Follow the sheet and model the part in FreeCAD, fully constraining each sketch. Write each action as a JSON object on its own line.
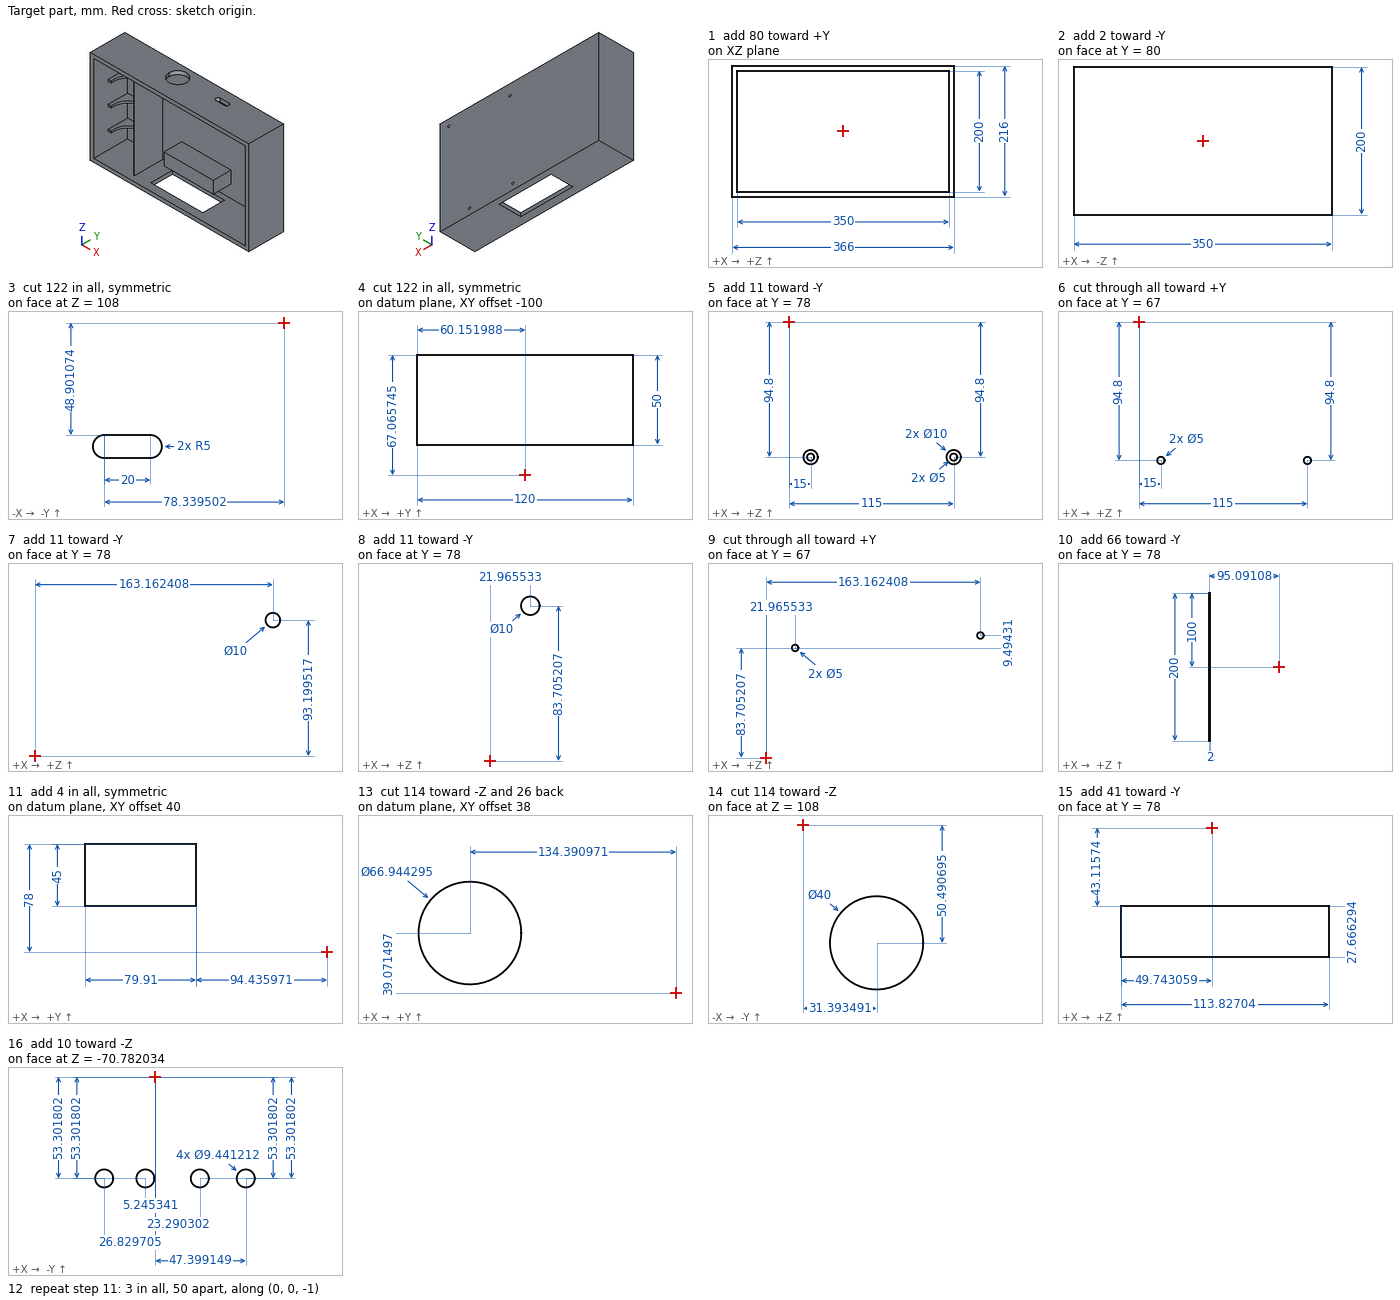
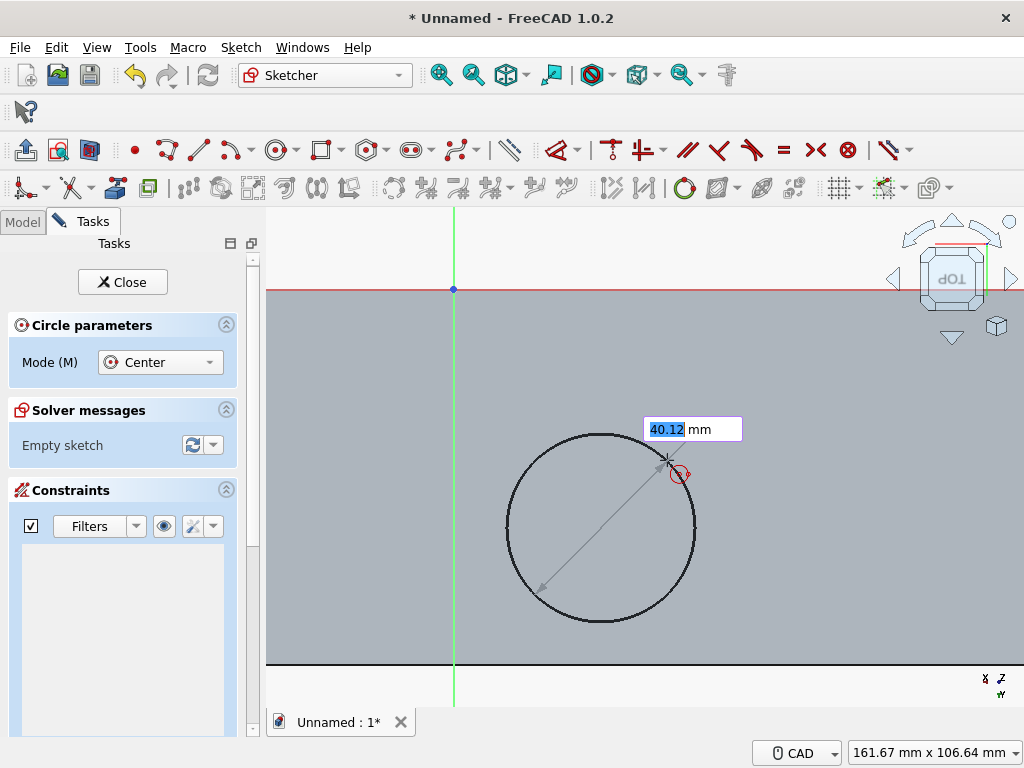
{"action": "type", "text": "40"}
{"action": "key", "text": "Return"}
{"action": "key", "text": "Escape"}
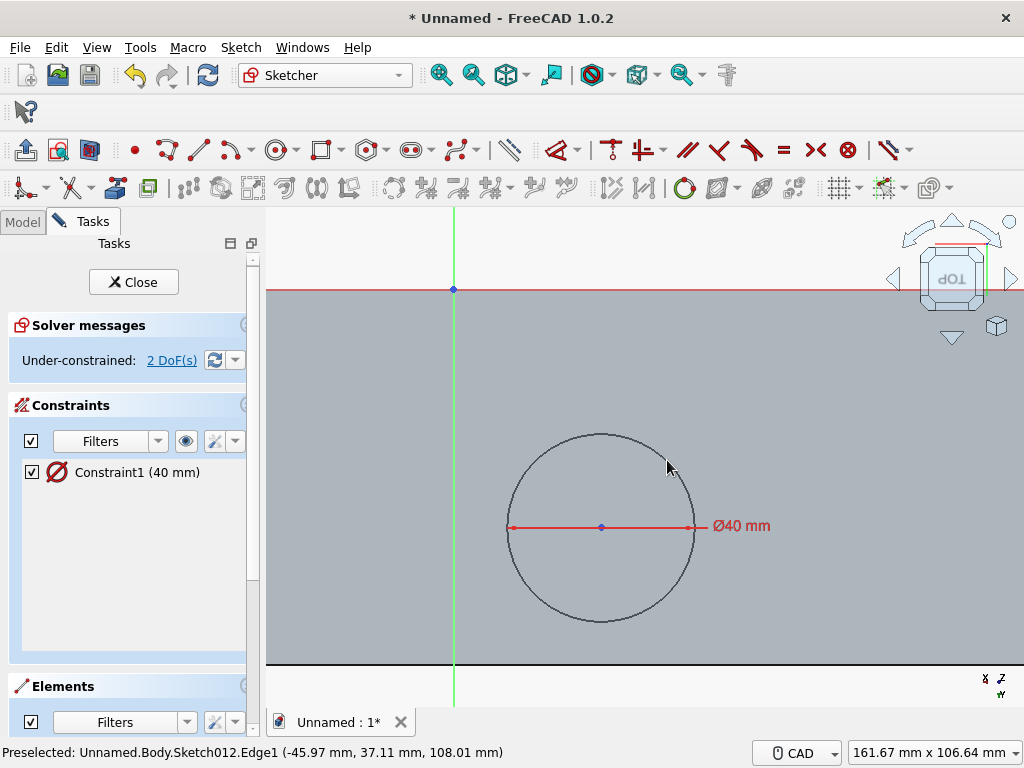
{"action": "left_click", "coordinate": [556, 150]}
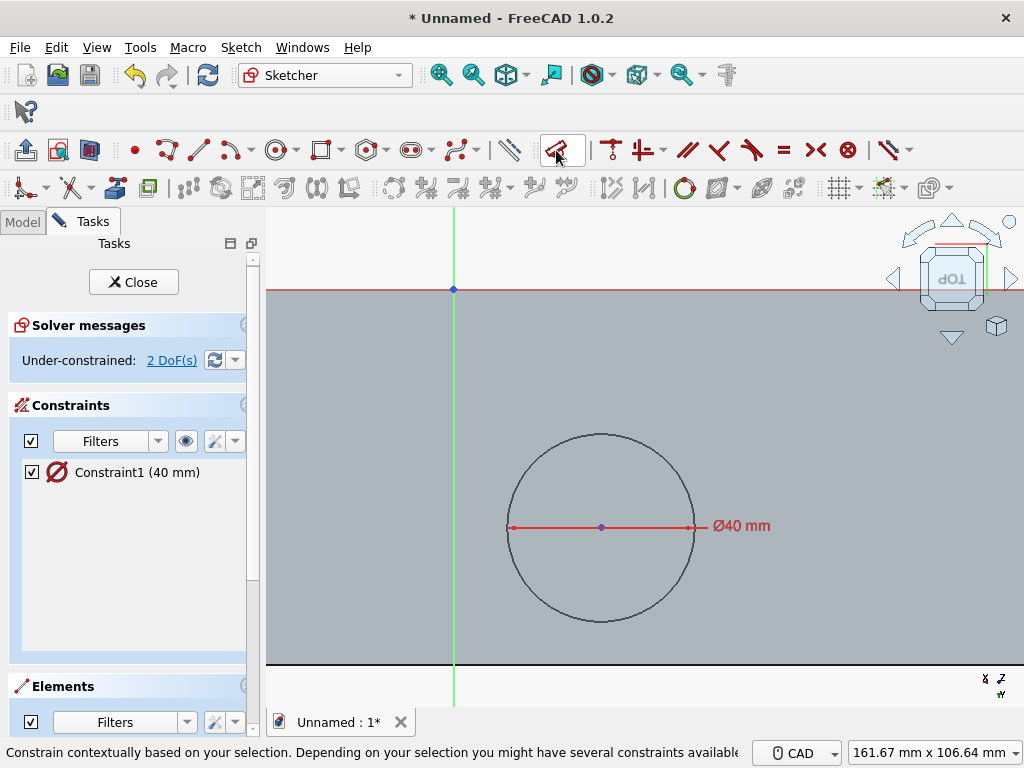
{"action": "left_click", "coordinate": [601, 528]}
{"action": "left_click", "coordinate": [527, 256]}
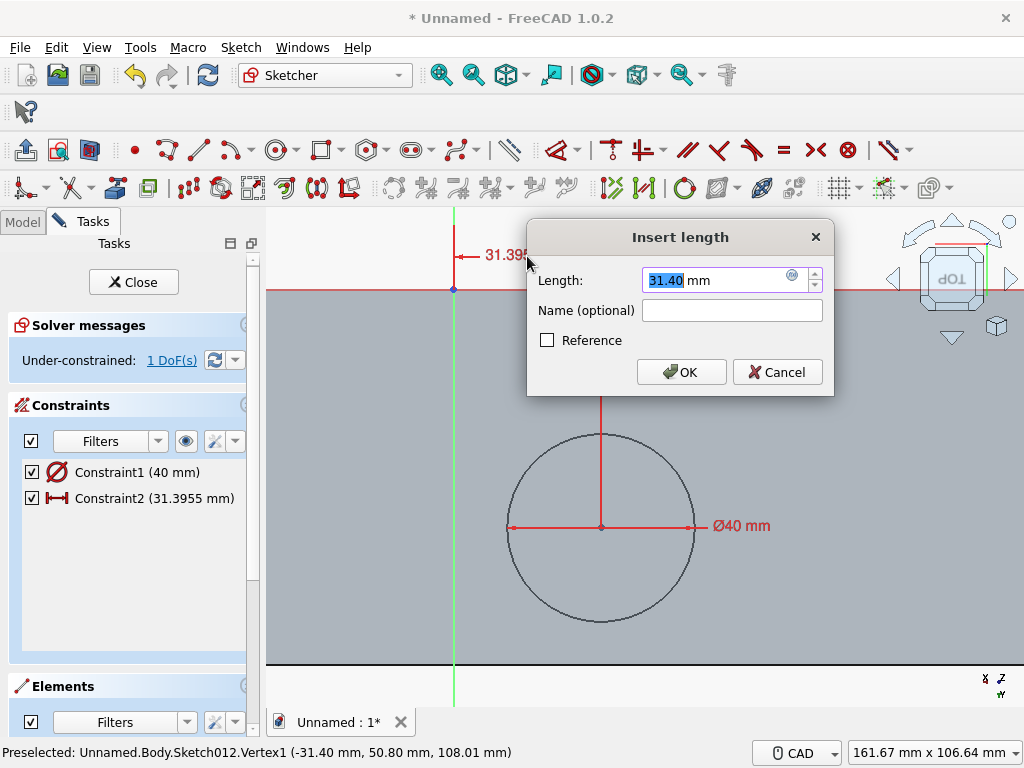
{"action": "type", "text": "31.393491"}
{"action": "key", "text": "Return"}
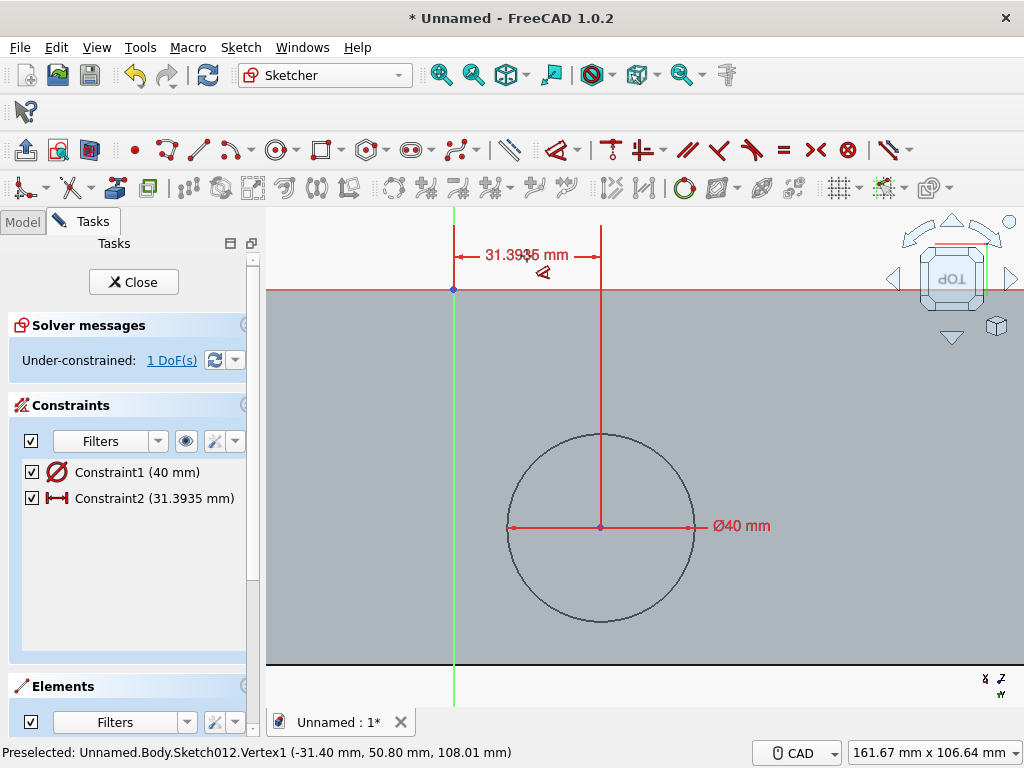
{"action": "left_click", "coordinate": [601, 528]}
{"action": "left_click", "coordinate": [420, 409]}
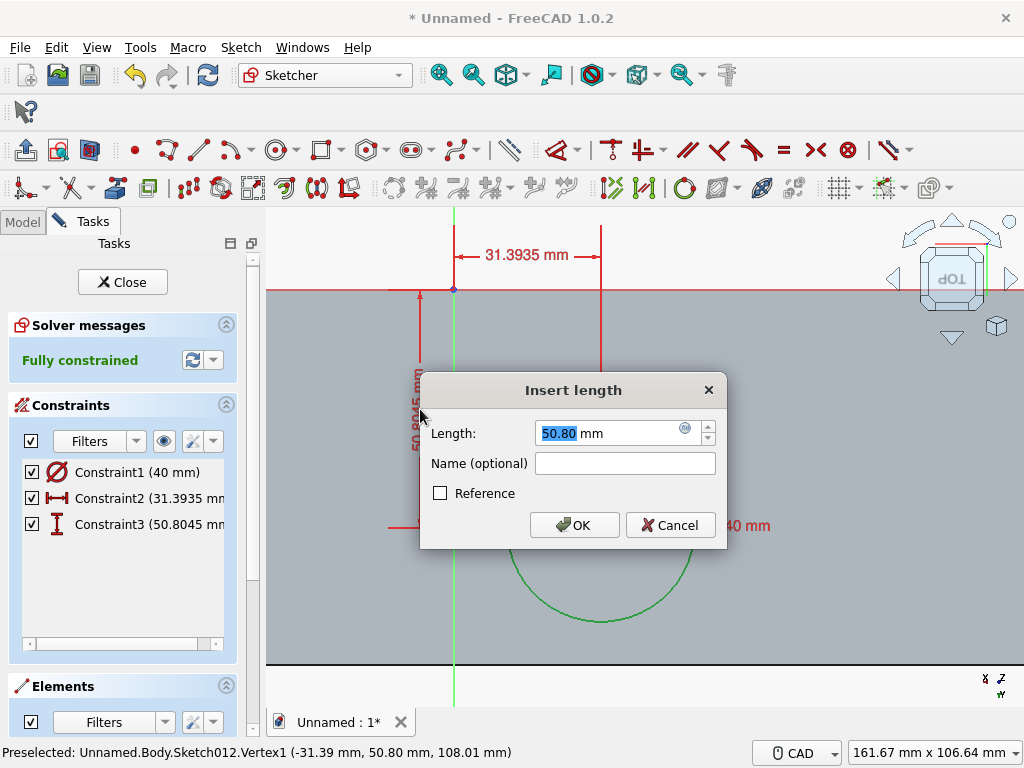
{"action": "type", "text": "50.490695"}
{"action": "key", "text": "Return"}
{"action": "key", "text": "Escape"}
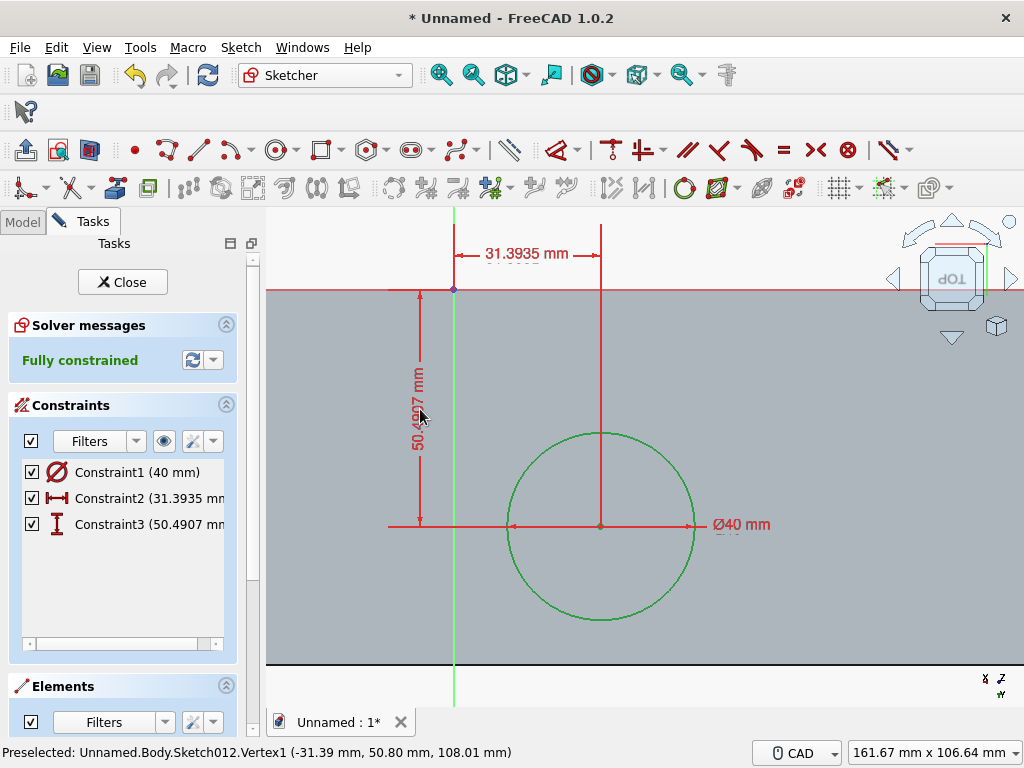
{"action": "left_click", "coordinate": [123, 282]}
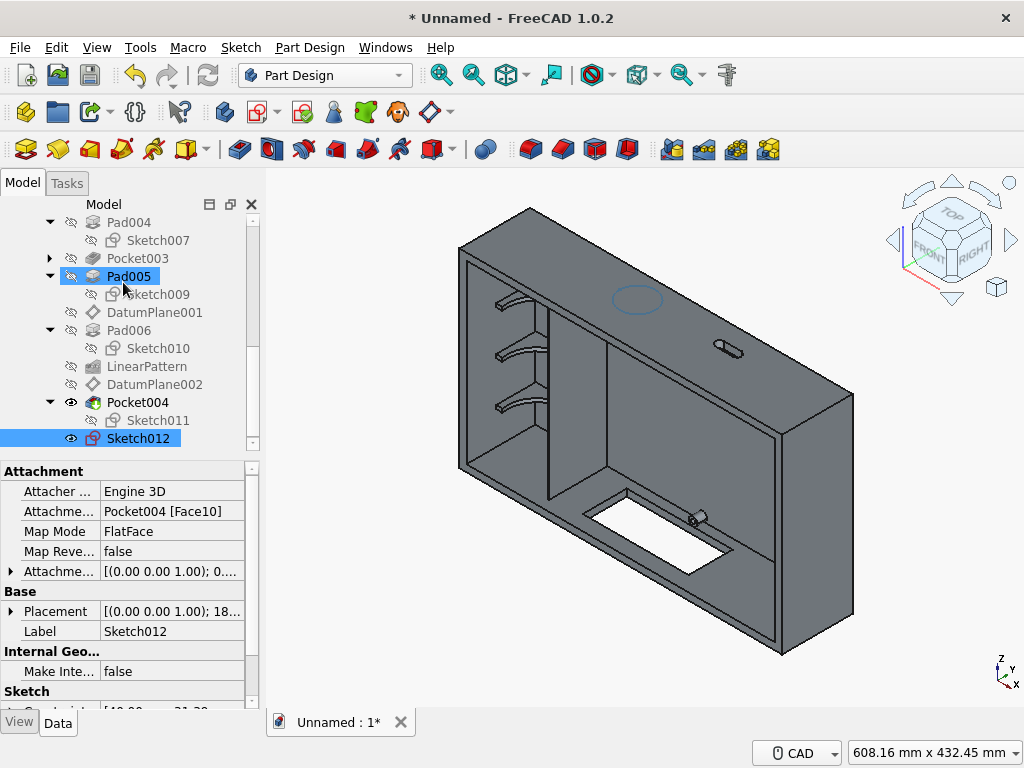
{"action": "left_click", "coordinate": [240, 150]}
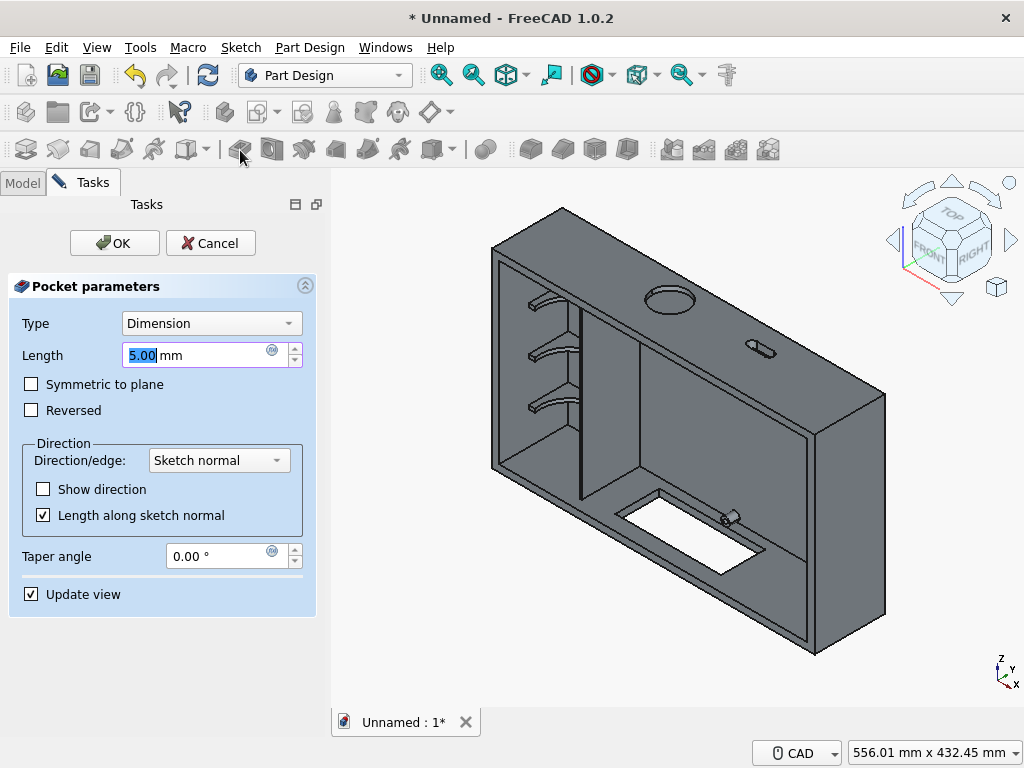
{"action": "type", "text": "114"}
{"action": "key", "text": "Tab"}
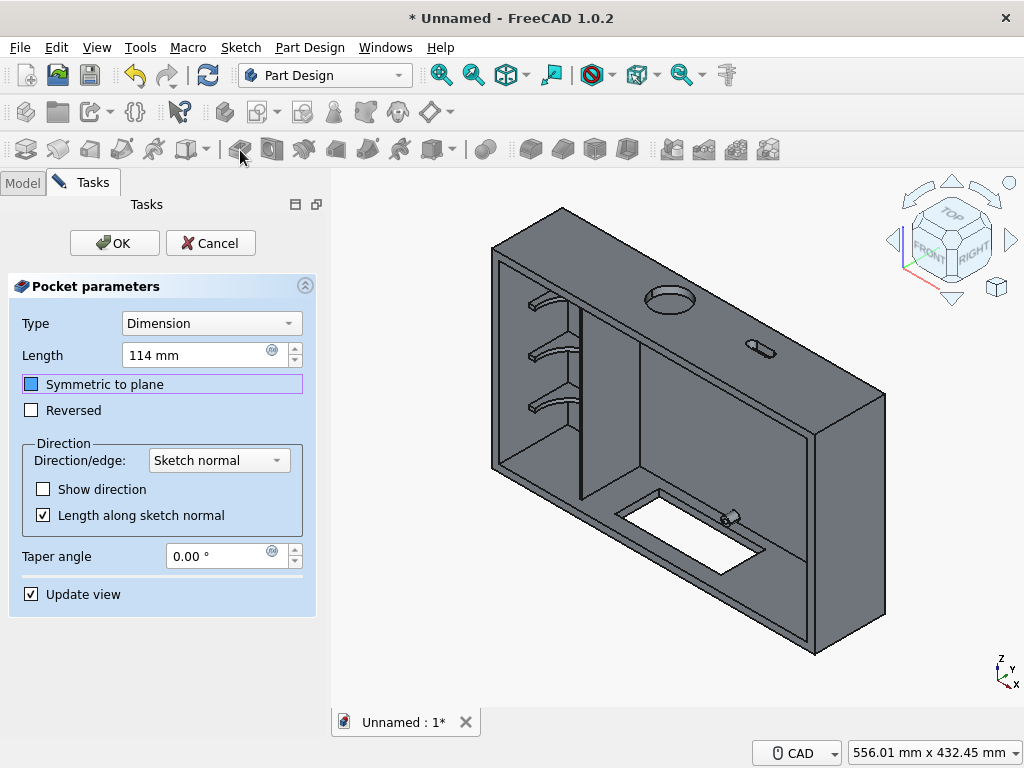
{"action": "left_click", "coordinate": [115, 243]}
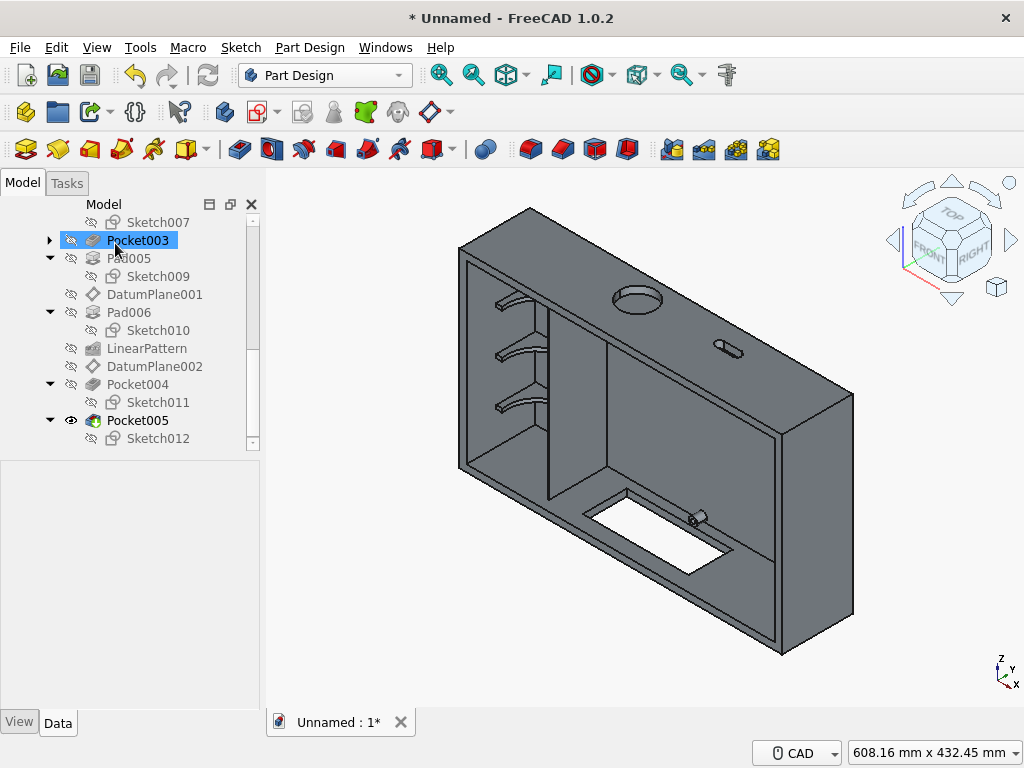
{"action": "left_click", "coordinate": [759, 451]}